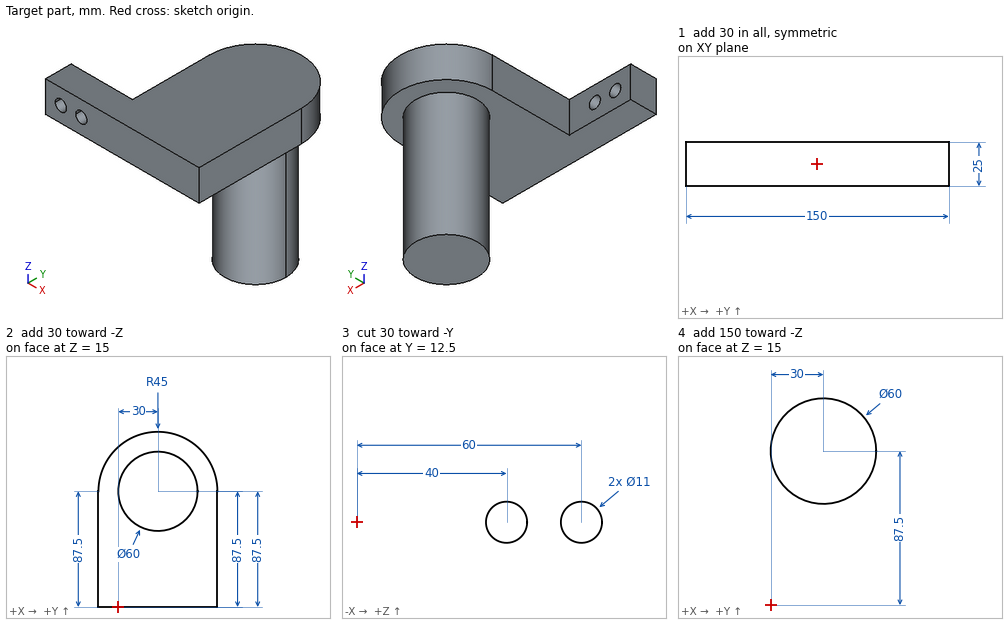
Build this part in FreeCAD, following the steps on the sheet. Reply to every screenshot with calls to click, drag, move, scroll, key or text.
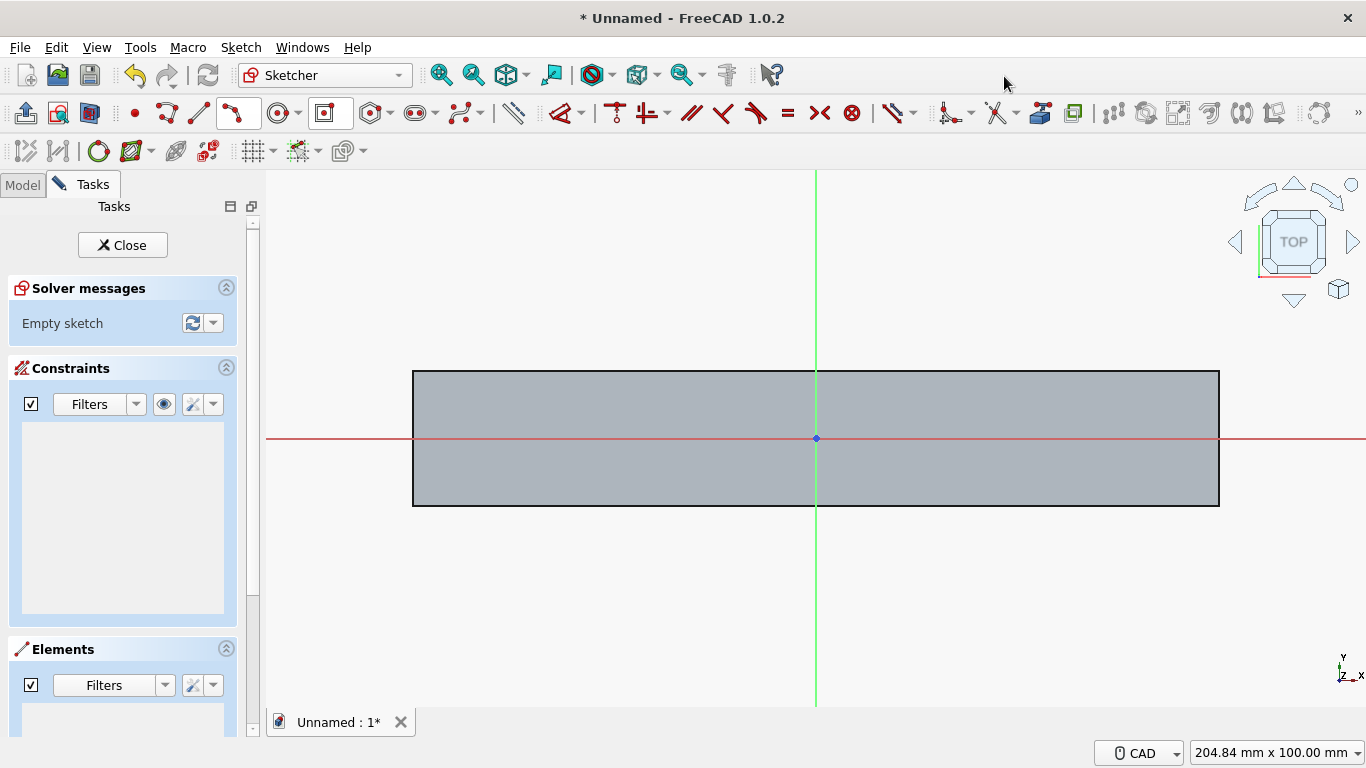
scroll(560, 679, down, 4)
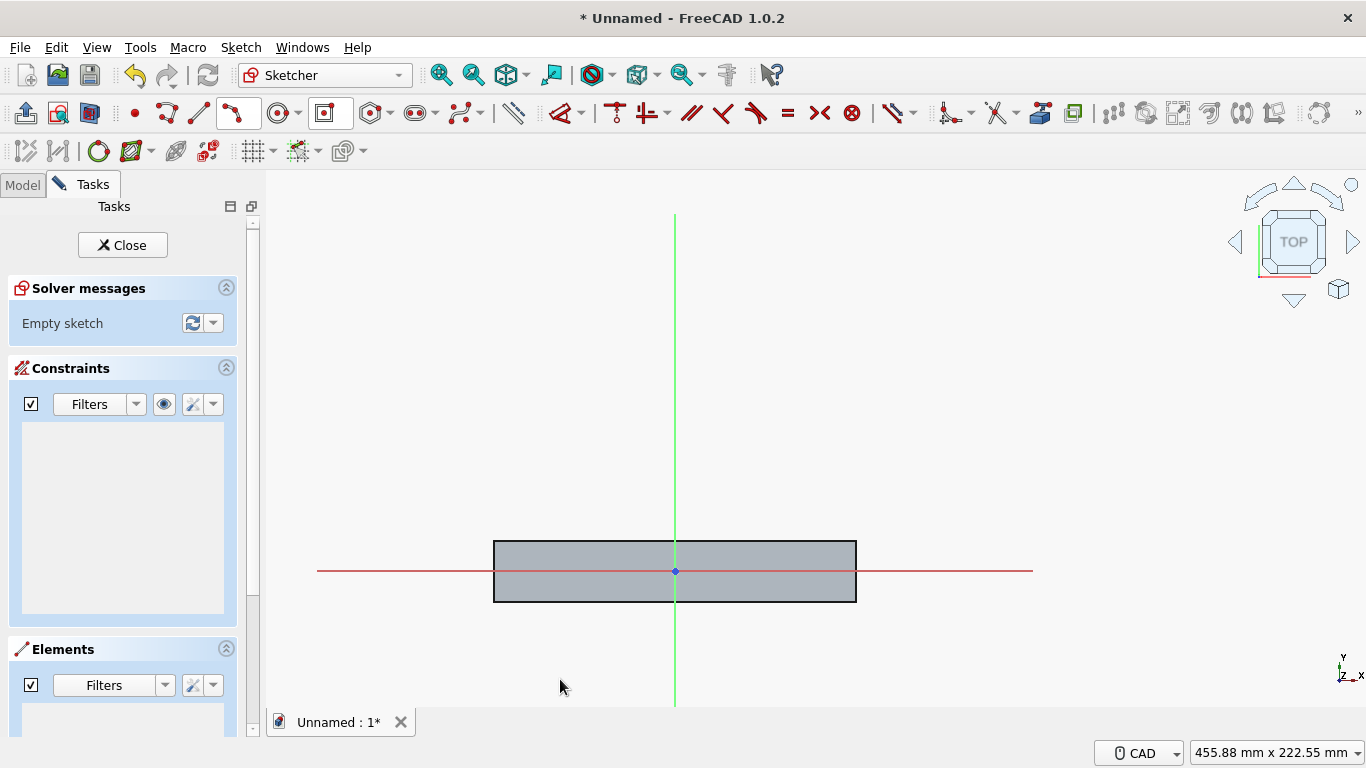
click(168, 114)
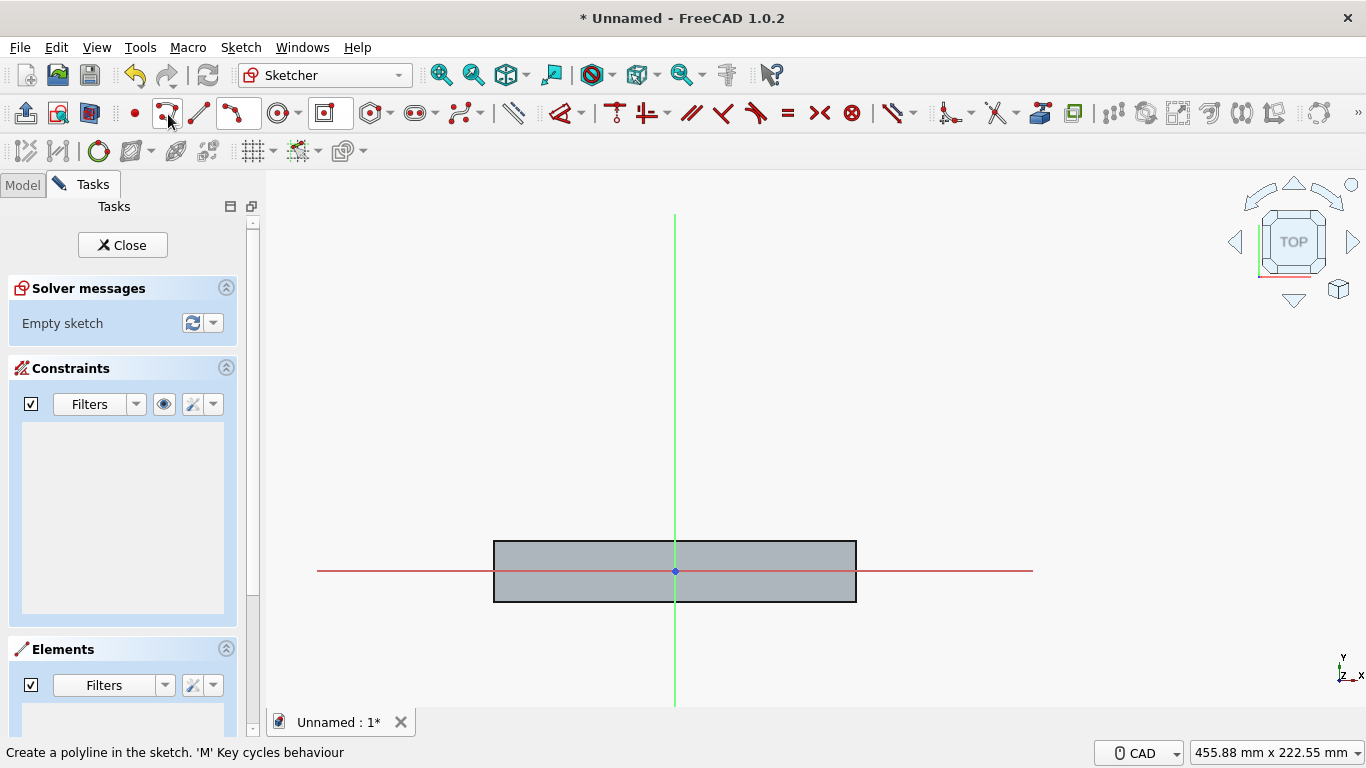
click(639, 360)
click(639, 571)
click(856, 562)
click(856, 360)
right_click(856, 360)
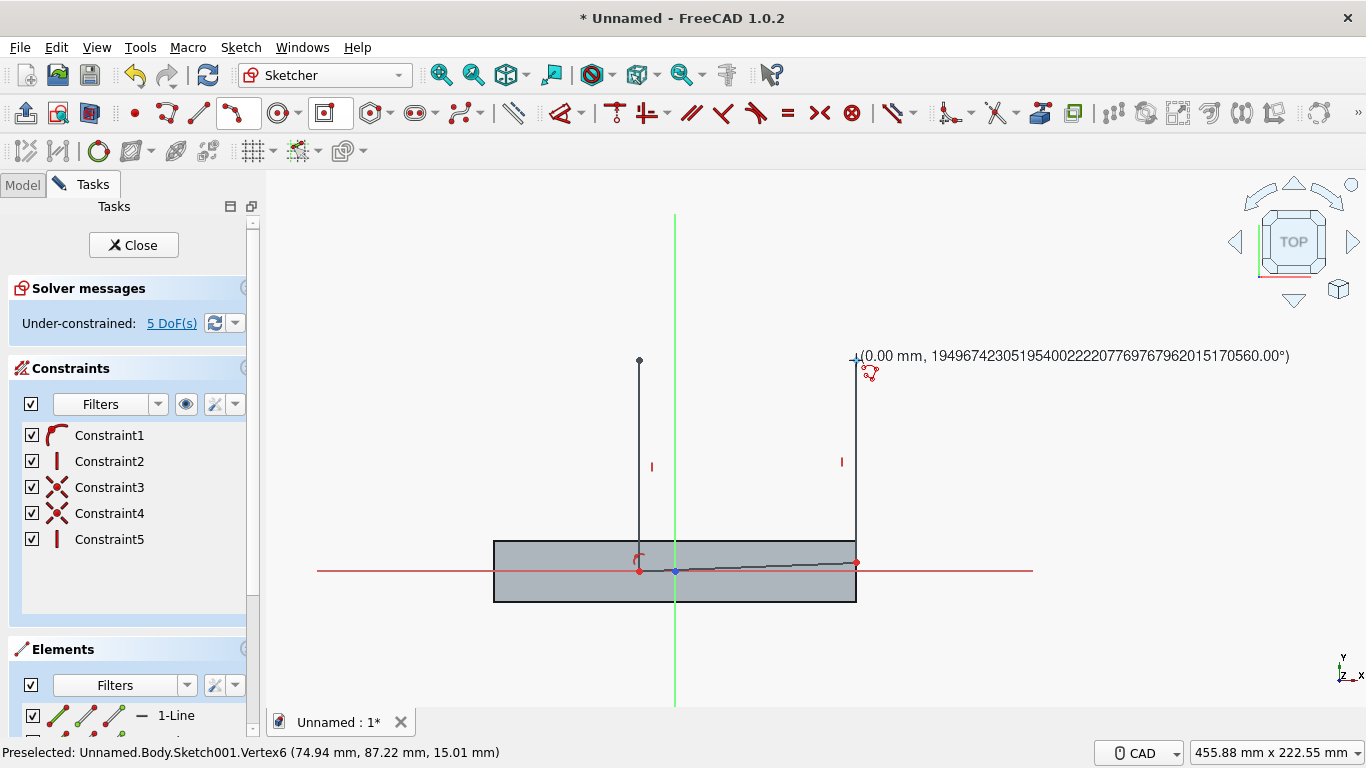
click(232, 114)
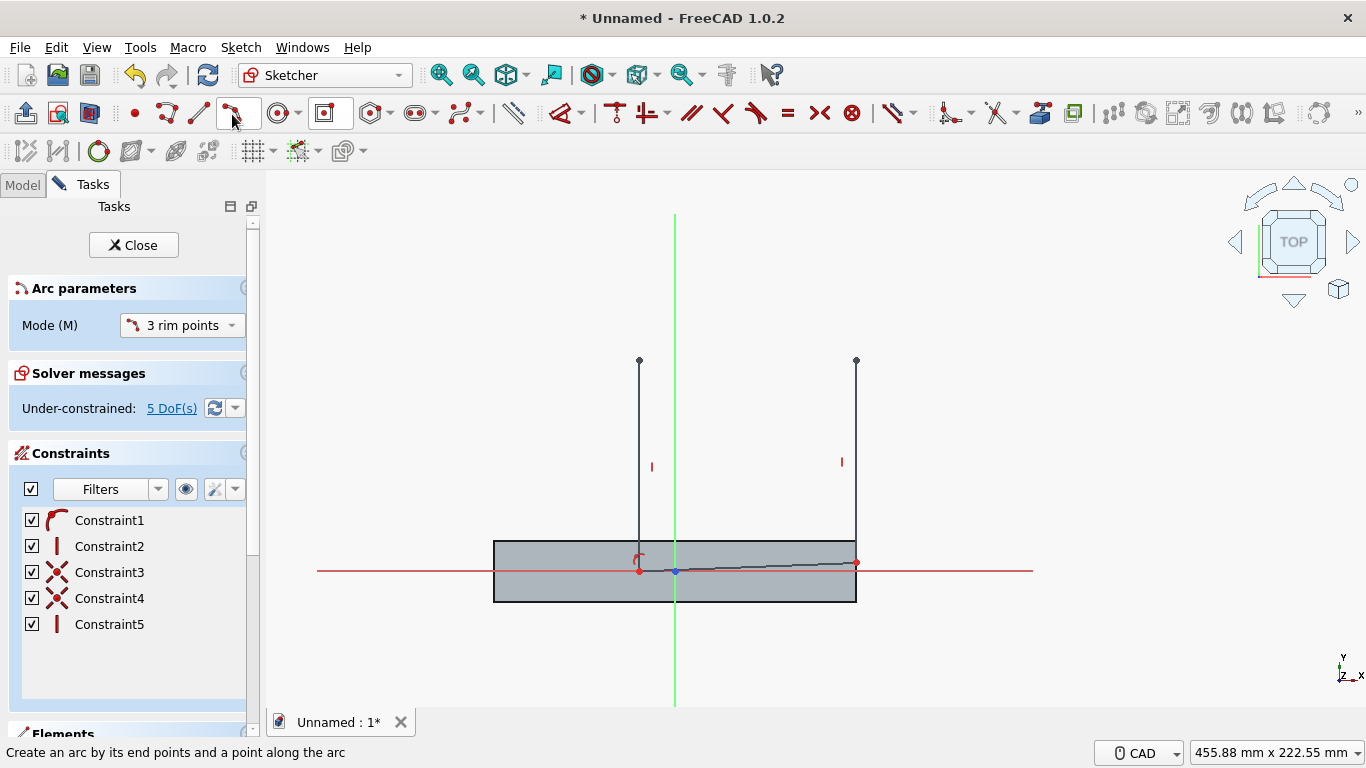
click(856, 361)
click(639, 361)
click(748, 252)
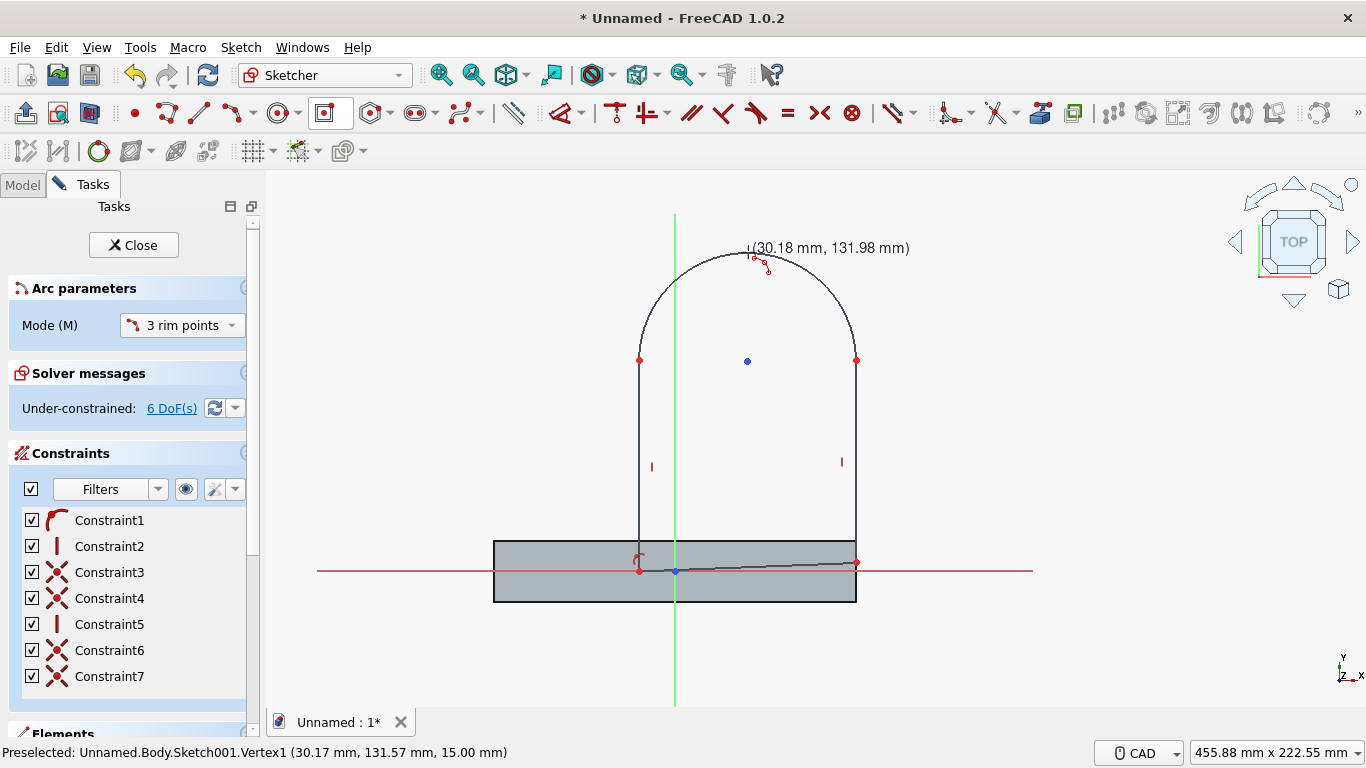
click(278, 114)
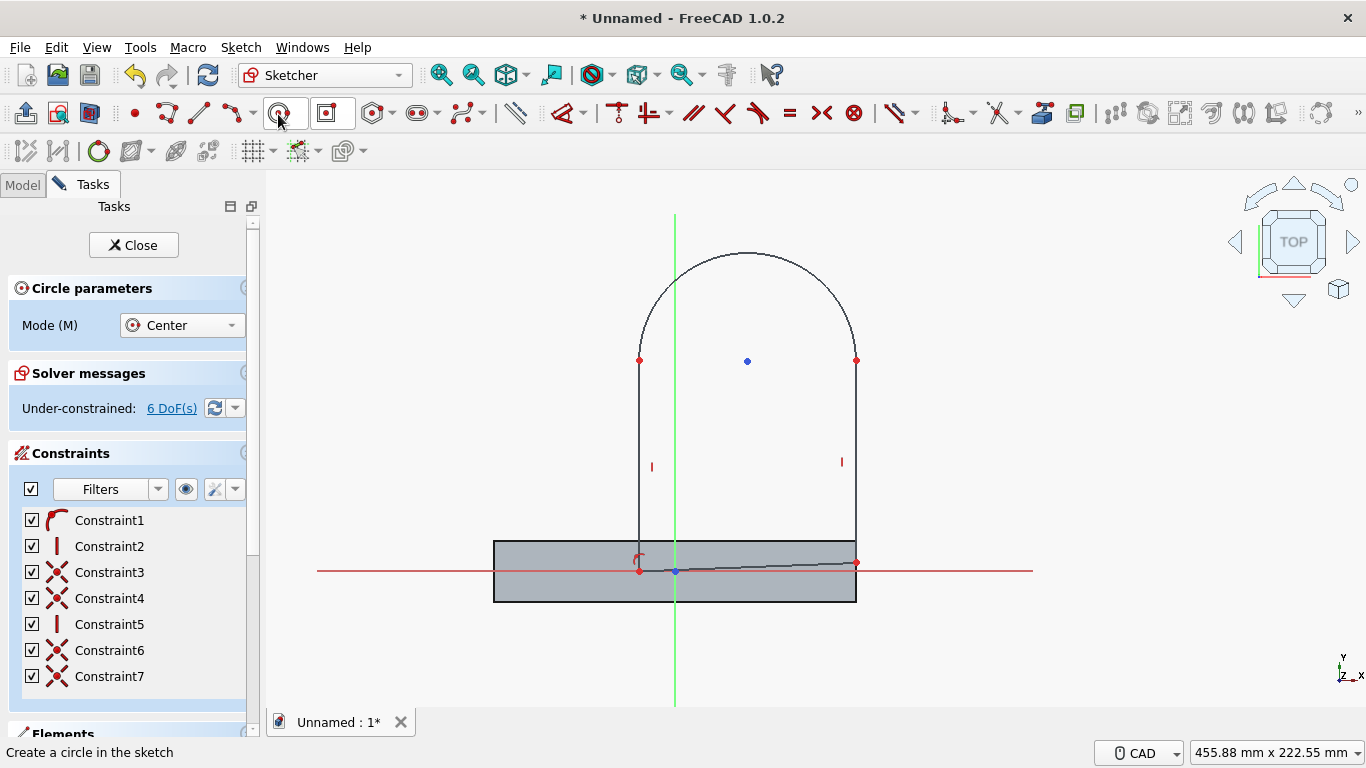
click(748, 360)
click(799, 309)
key(Escape)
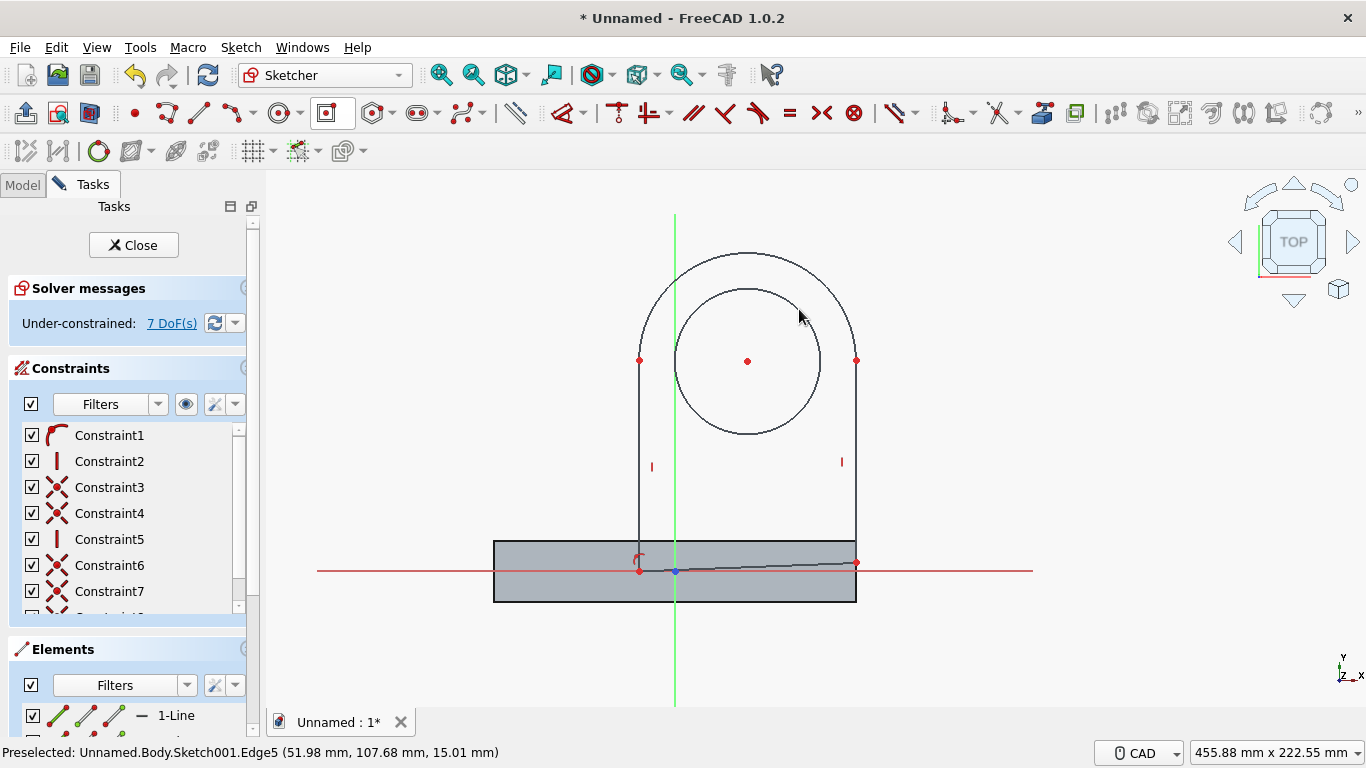
click(704, 569)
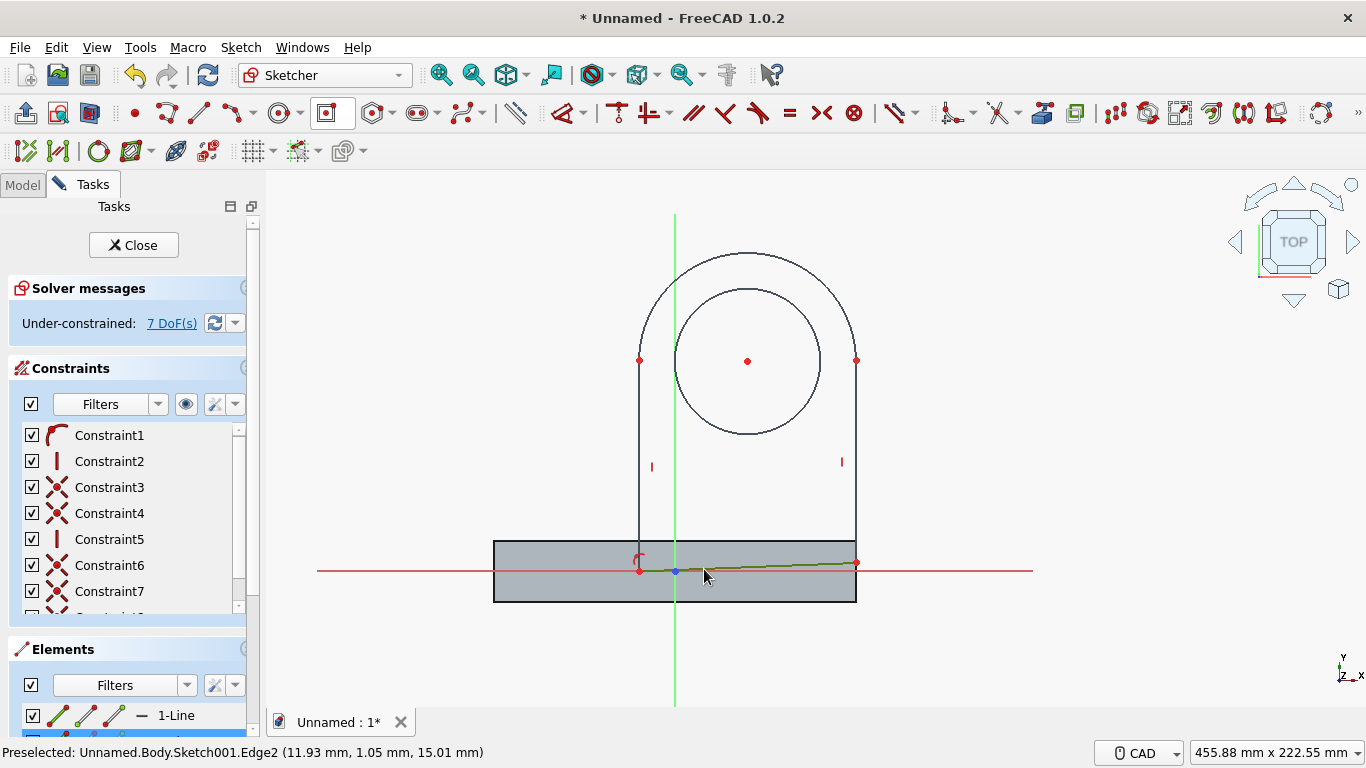
key(h)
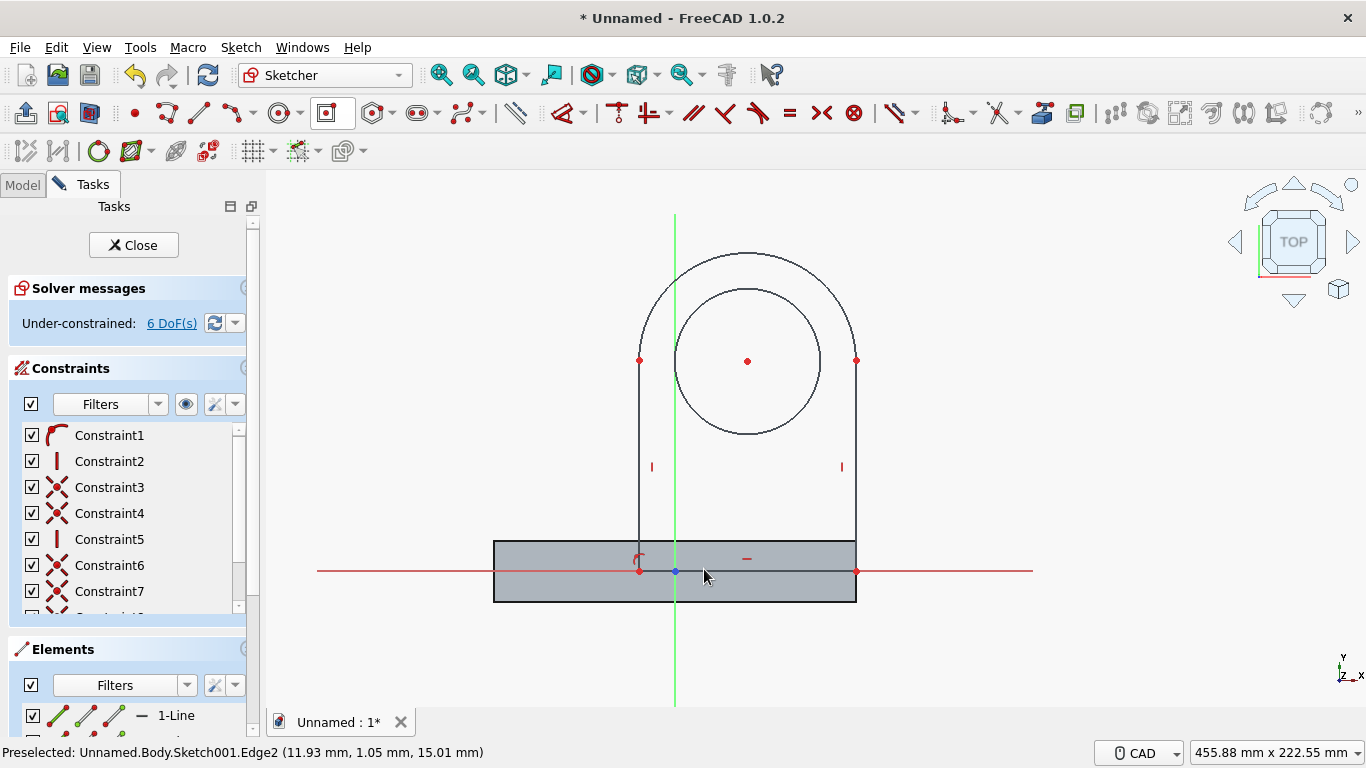
click(562, 114)